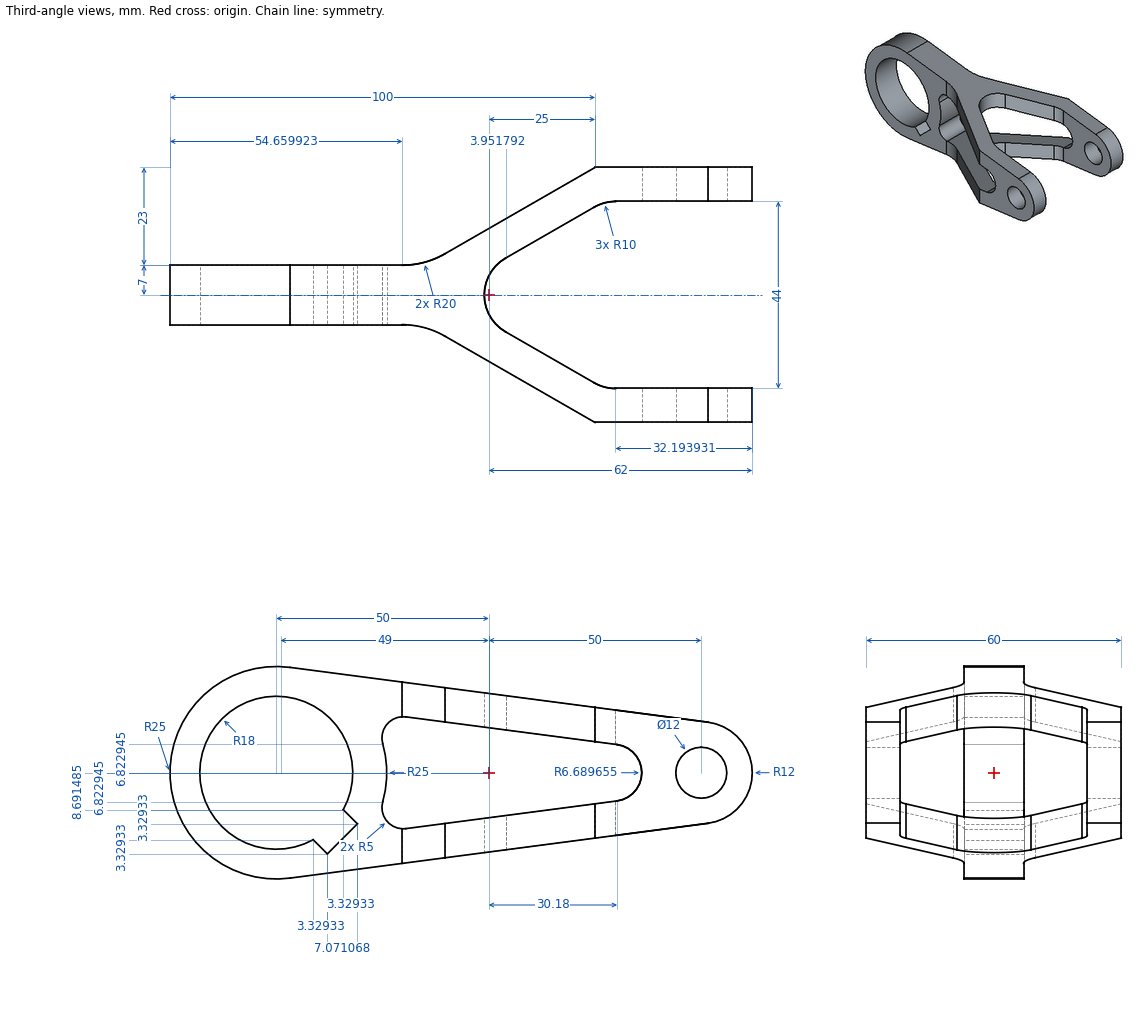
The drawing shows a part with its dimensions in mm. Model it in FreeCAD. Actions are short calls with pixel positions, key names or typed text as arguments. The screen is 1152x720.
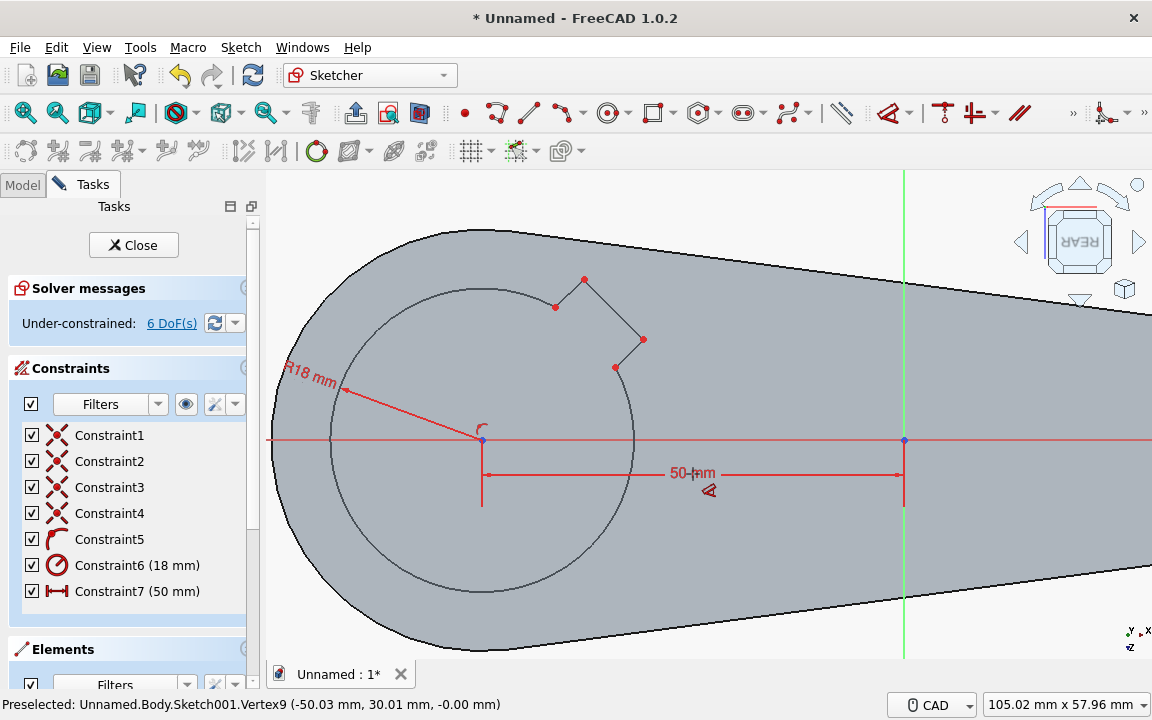
scroll(624, 360, up, 2)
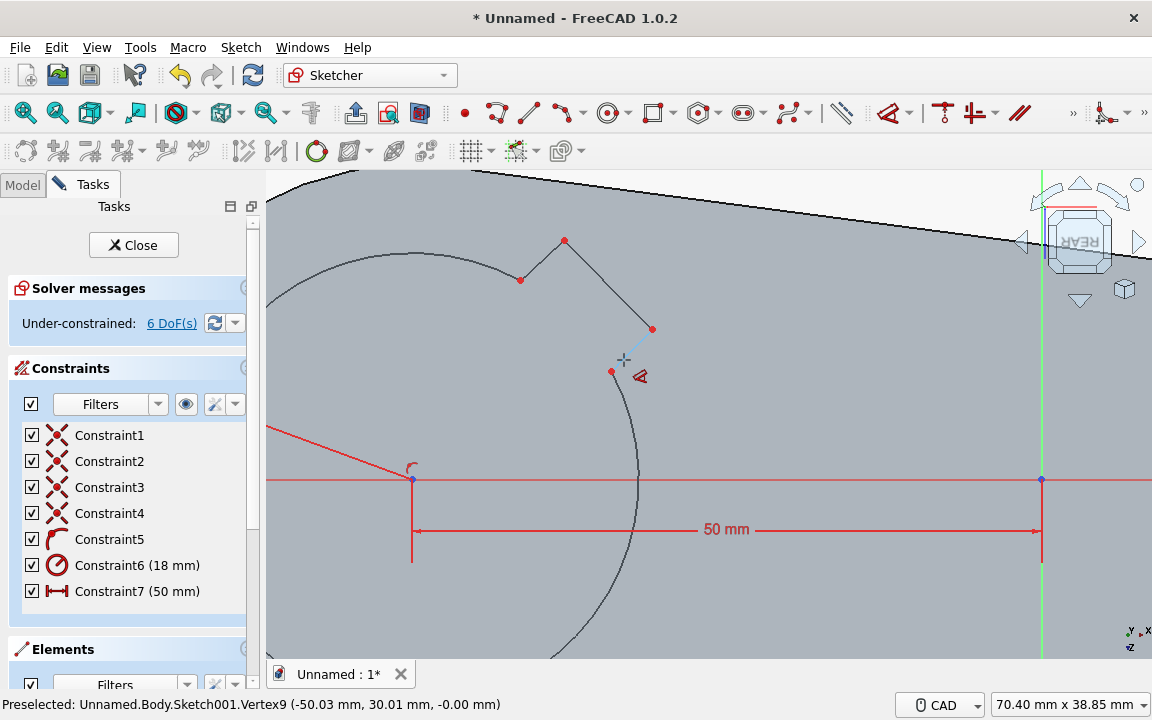
click(624, 359)
click(641, 296)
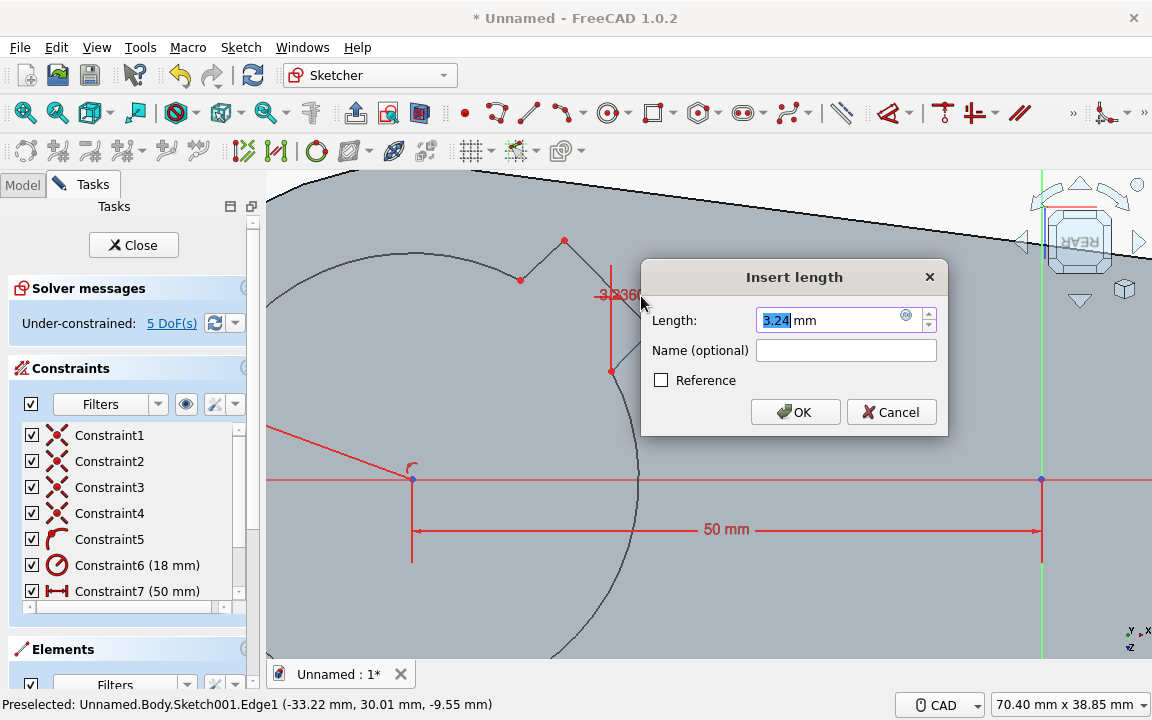
text(3.32933)
key(Return)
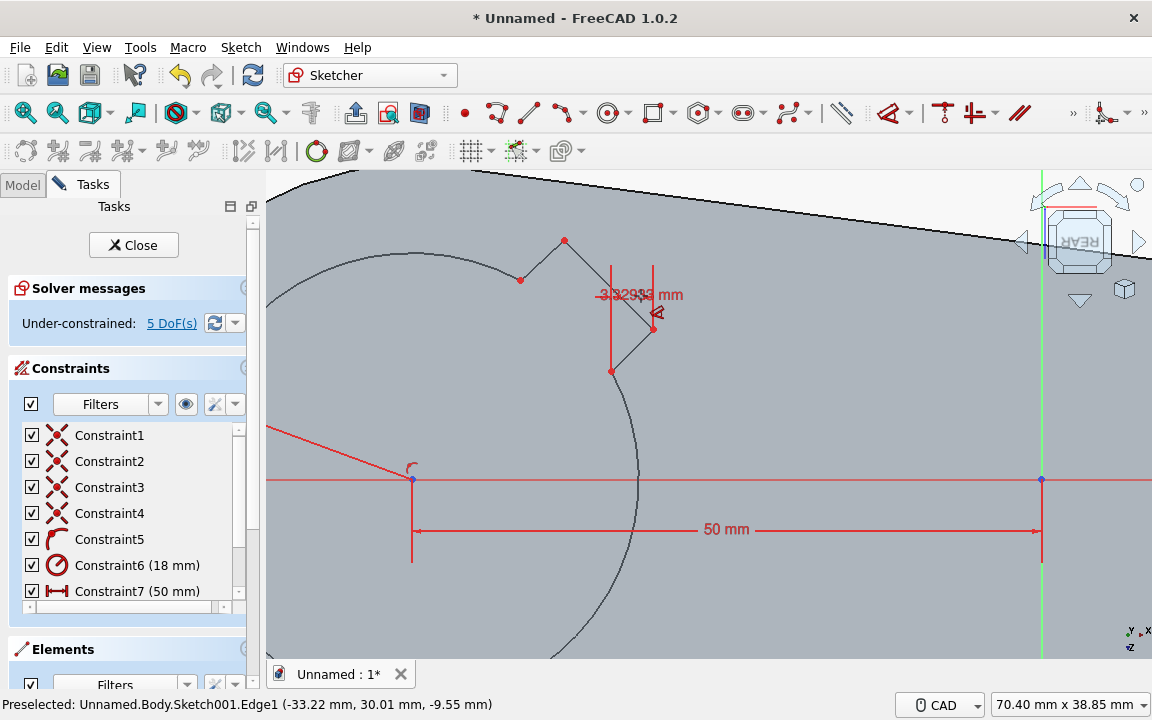
click(624, 359)
click(577, 351)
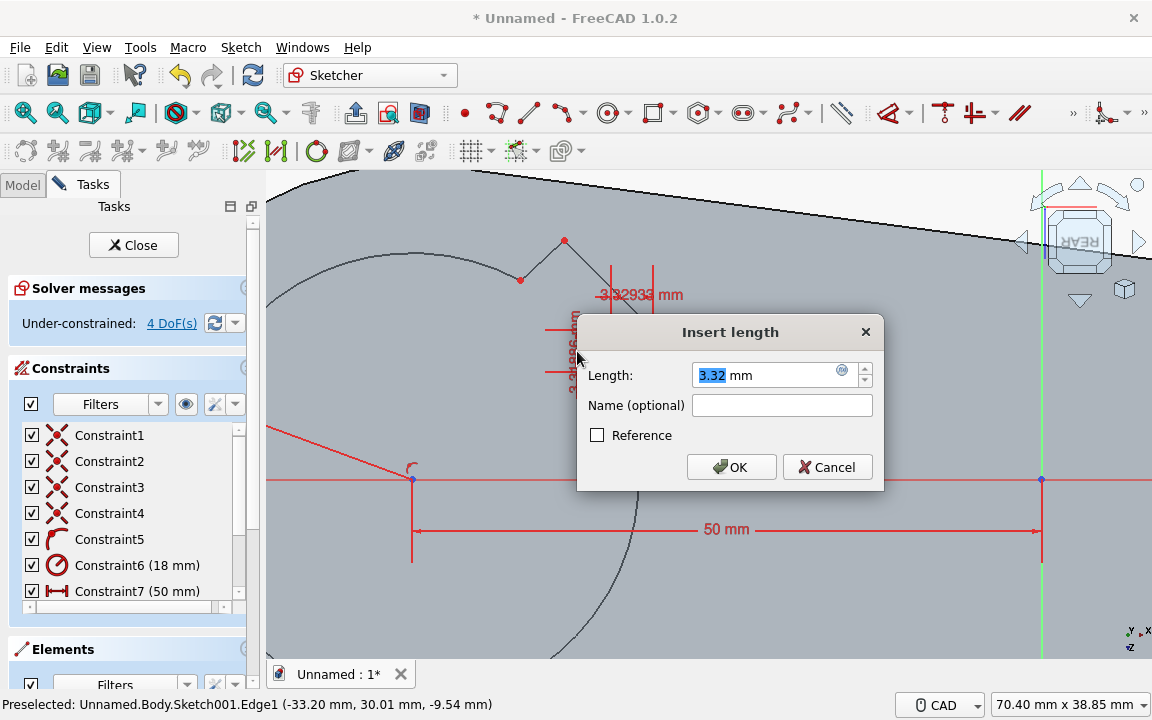
text(3.32933)
key(Return)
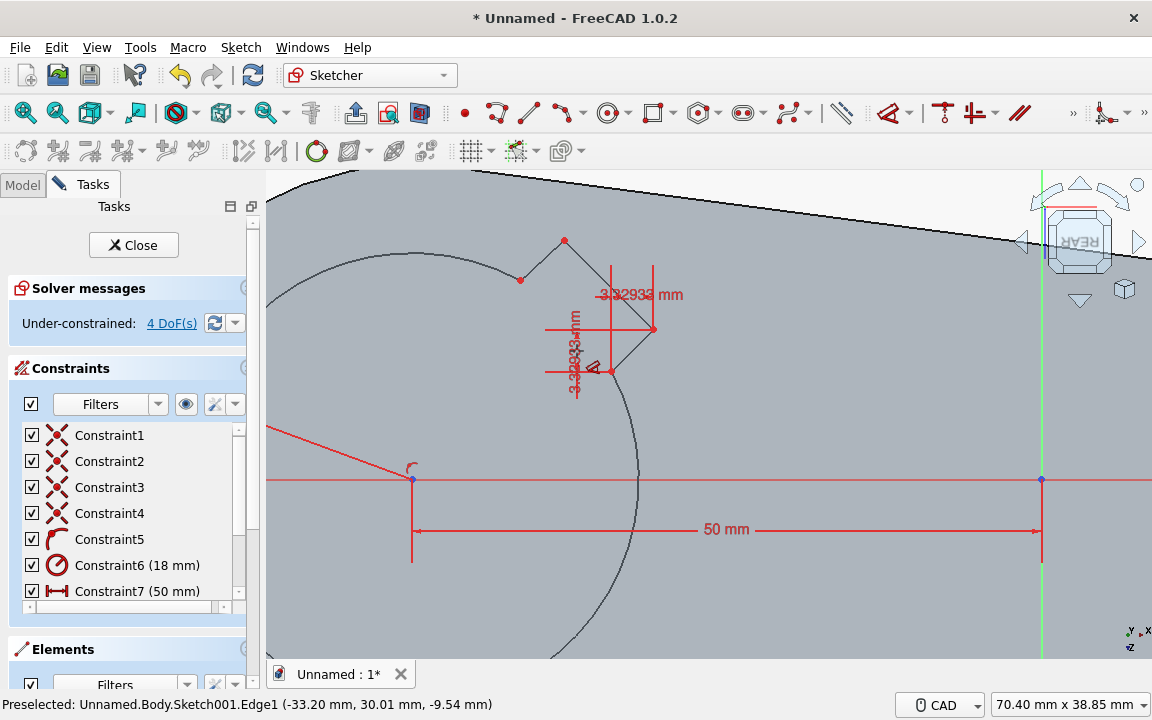
click(551, 253)
click(542, 206)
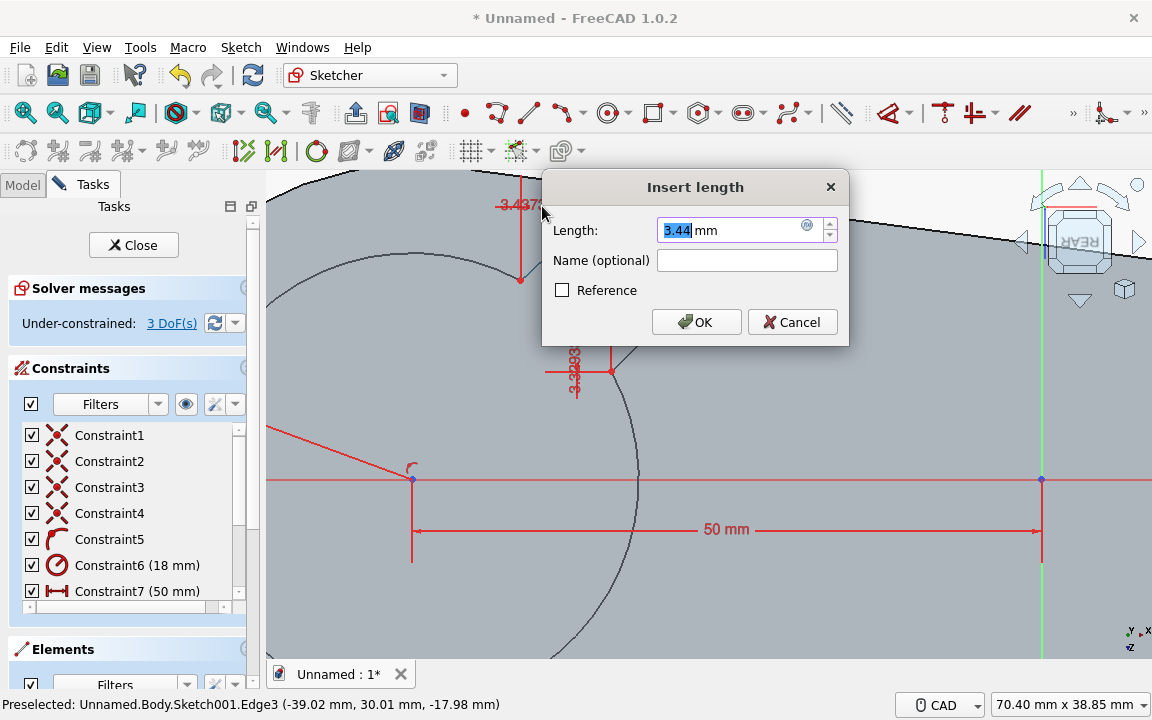
text(3.32933)
key(Return)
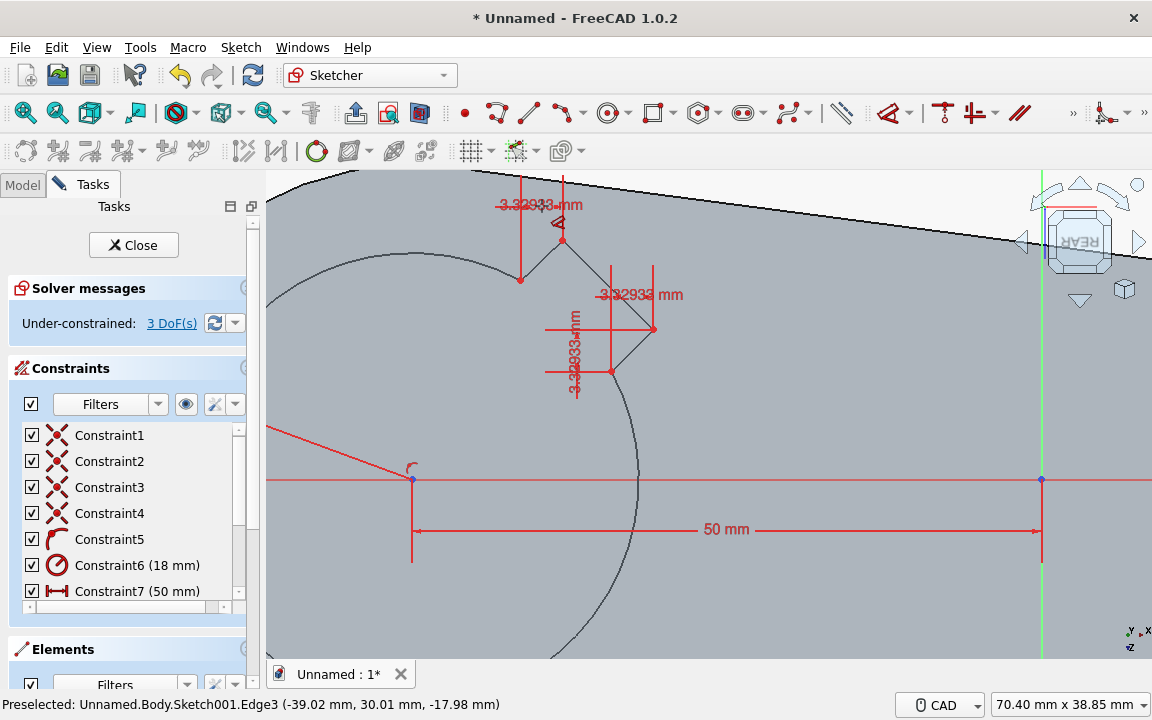
click(550, 253)
click(487, 251)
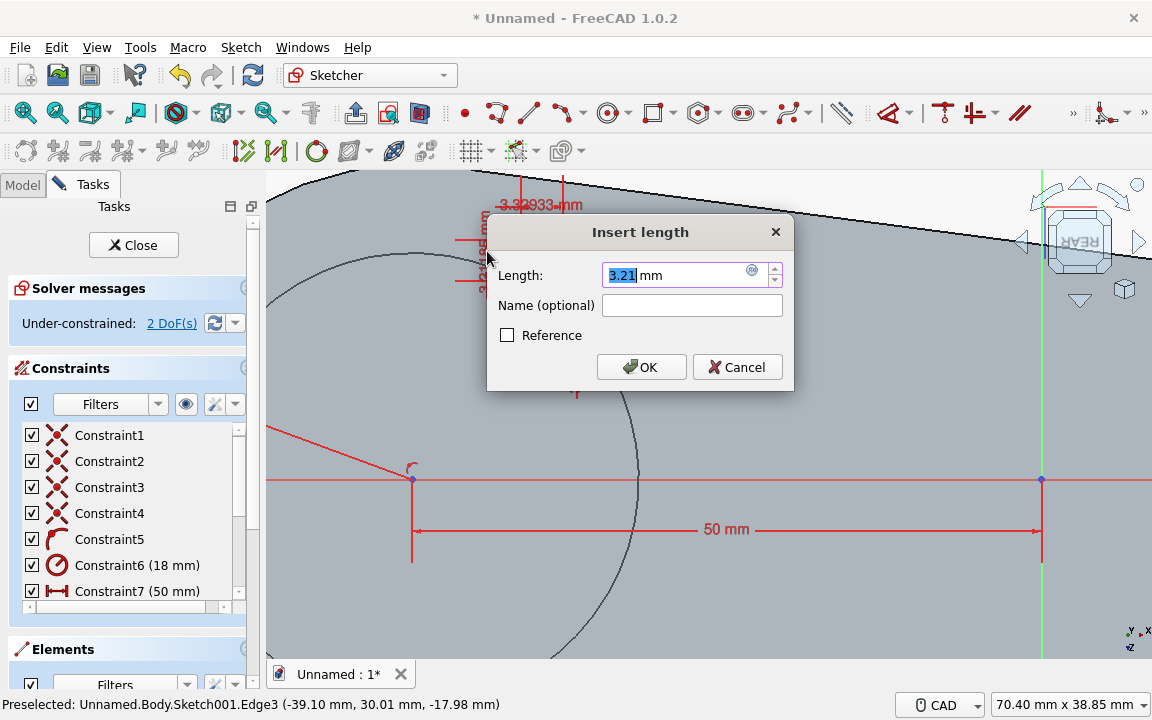
text(3.32933)
key(Return)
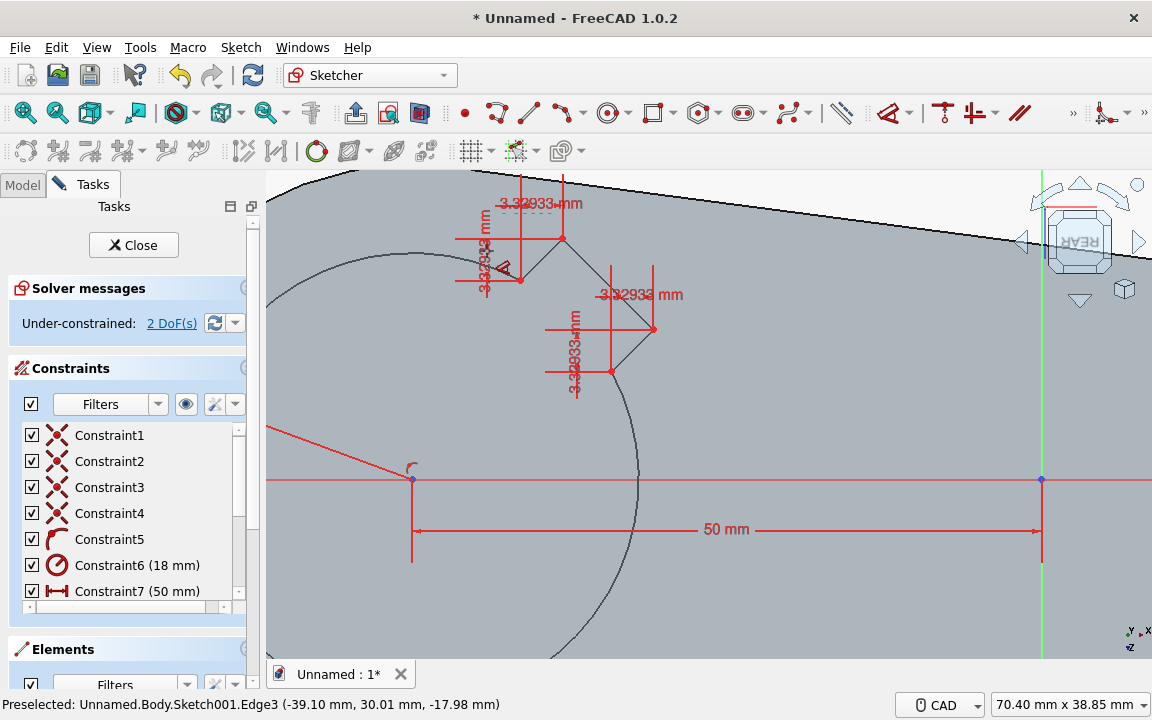
click(611, 372)
click(577, 426)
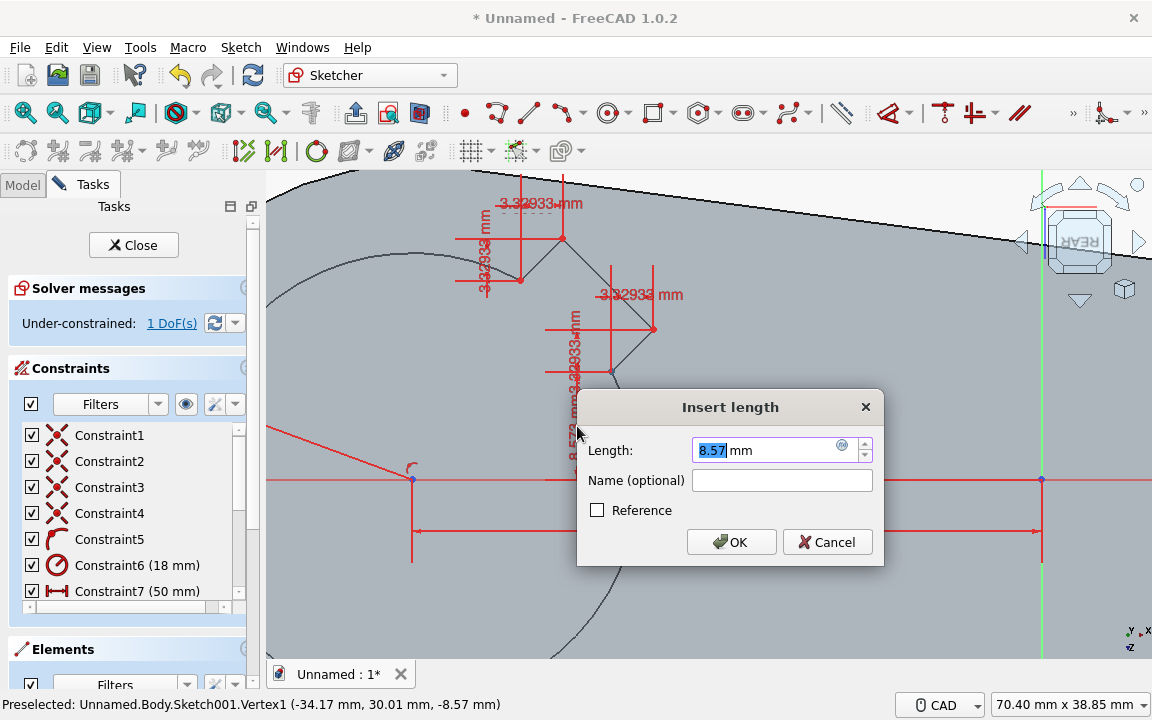
text(8.691485)
key(Return)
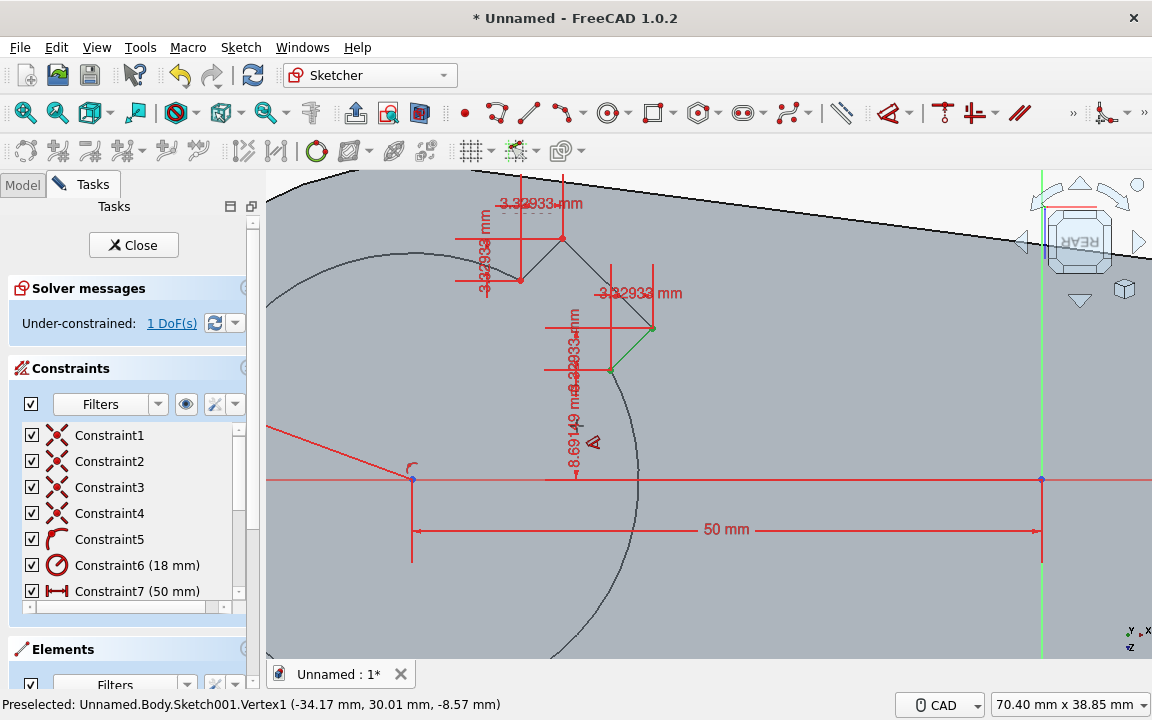
click(626, 302)
click(628, 205)